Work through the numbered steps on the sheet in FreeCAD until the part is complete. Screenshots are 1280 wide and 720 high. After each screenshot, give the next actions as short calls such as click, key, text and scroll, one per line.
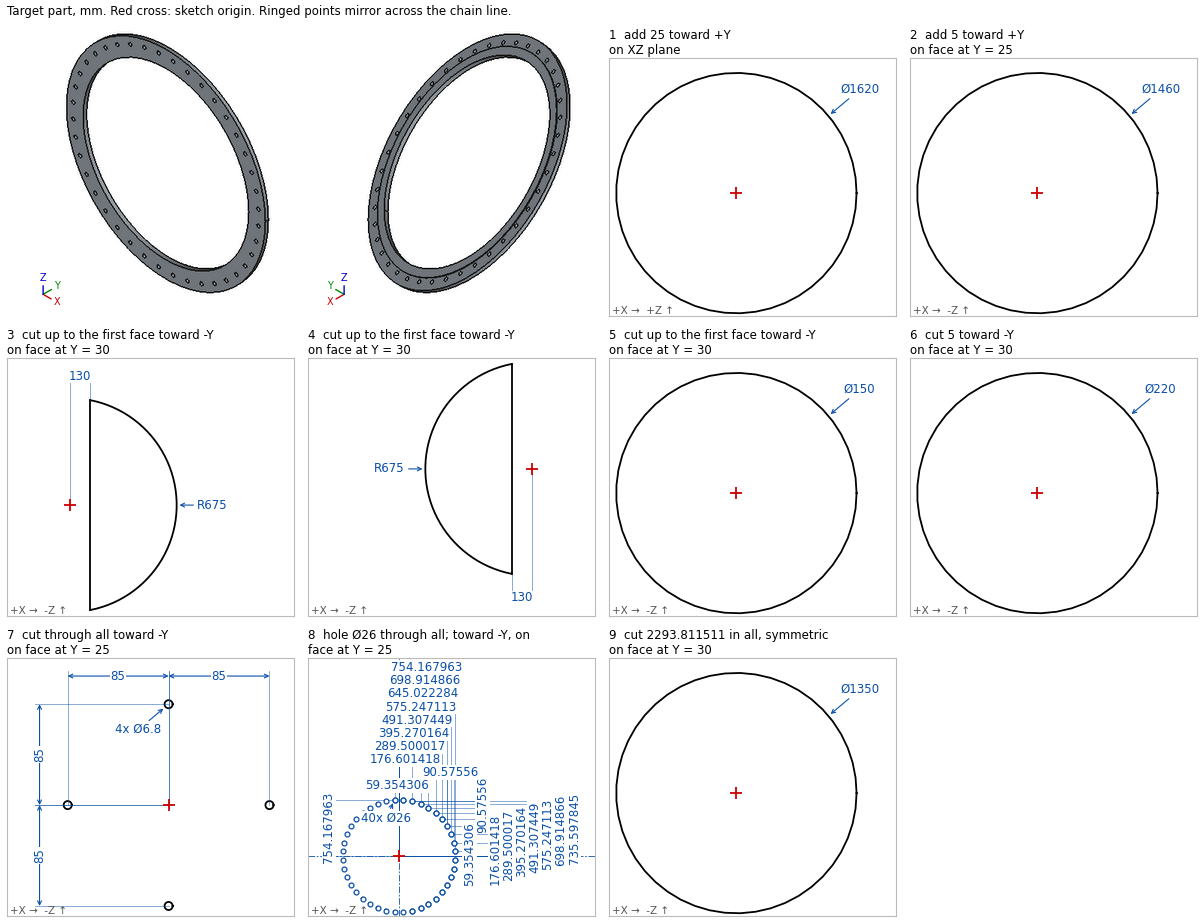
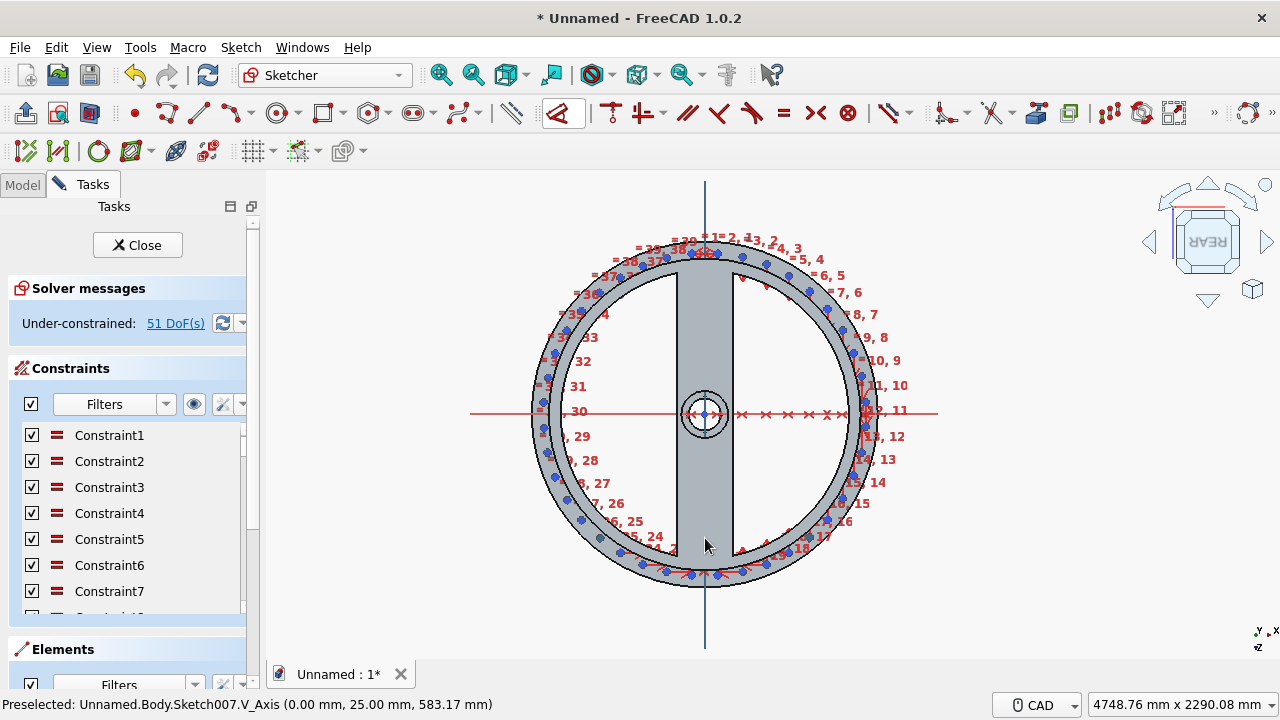
click(816, 114)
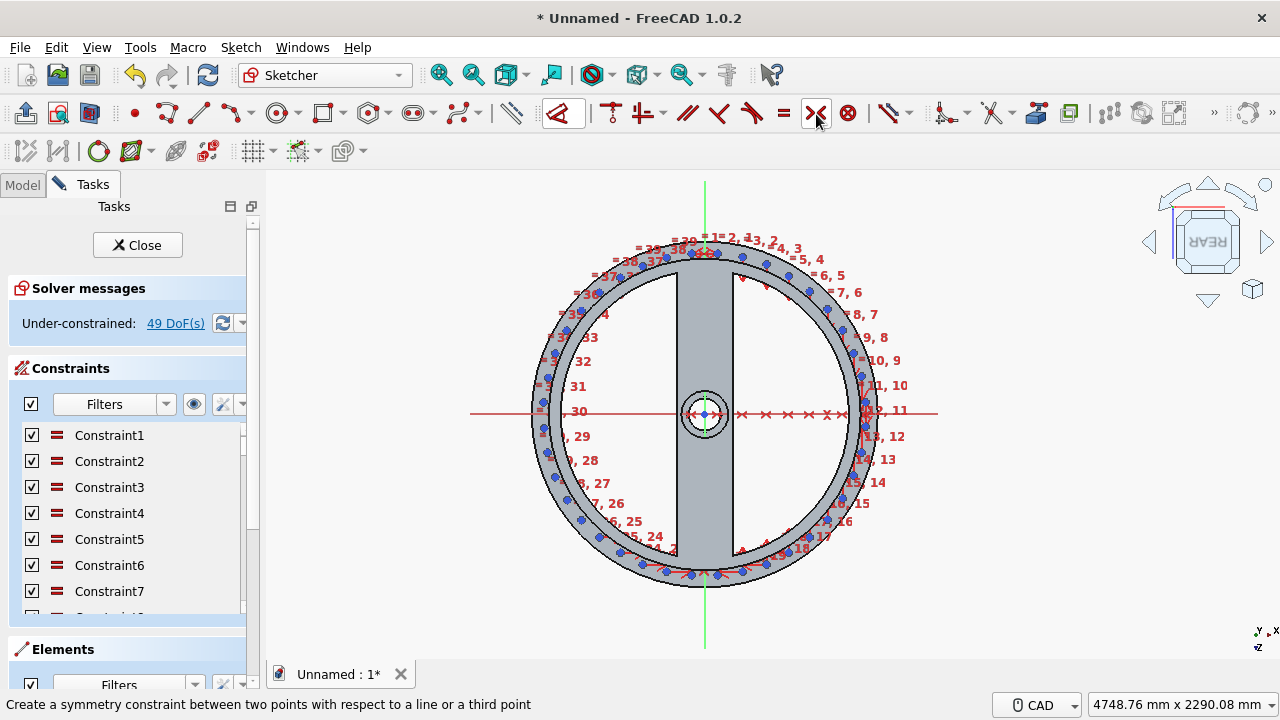
click(828, 520)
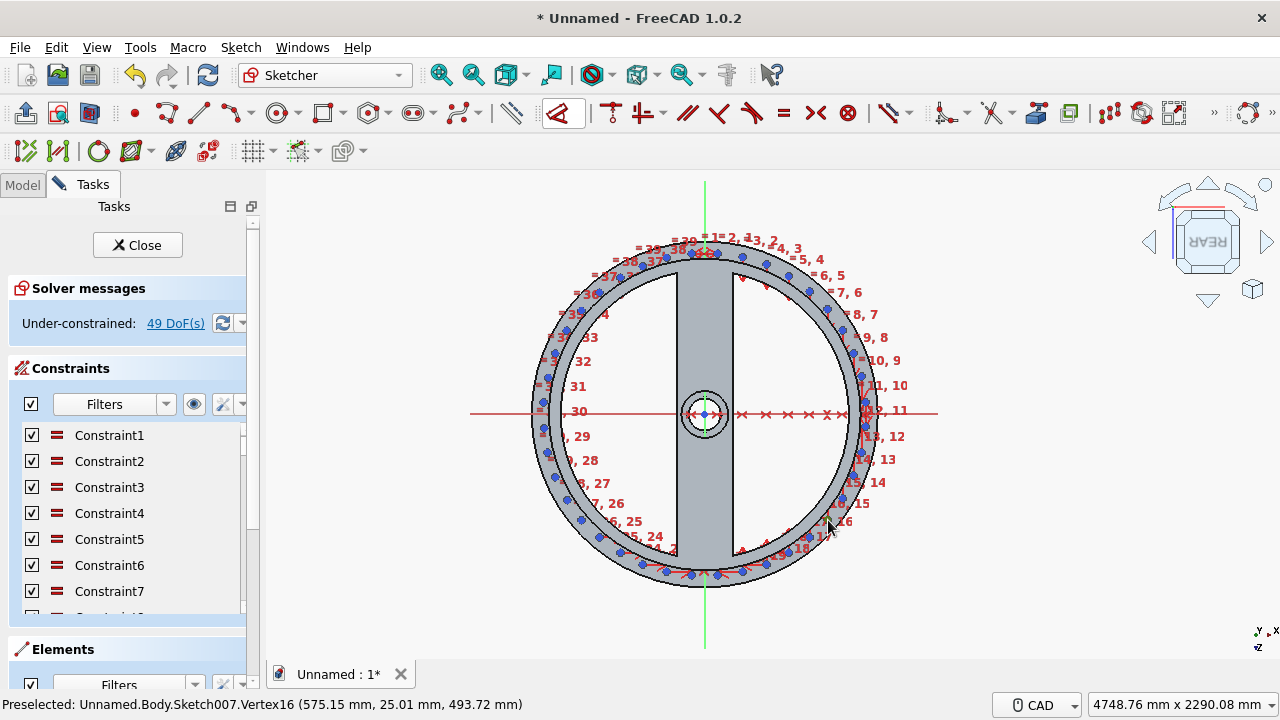
click(582, 520)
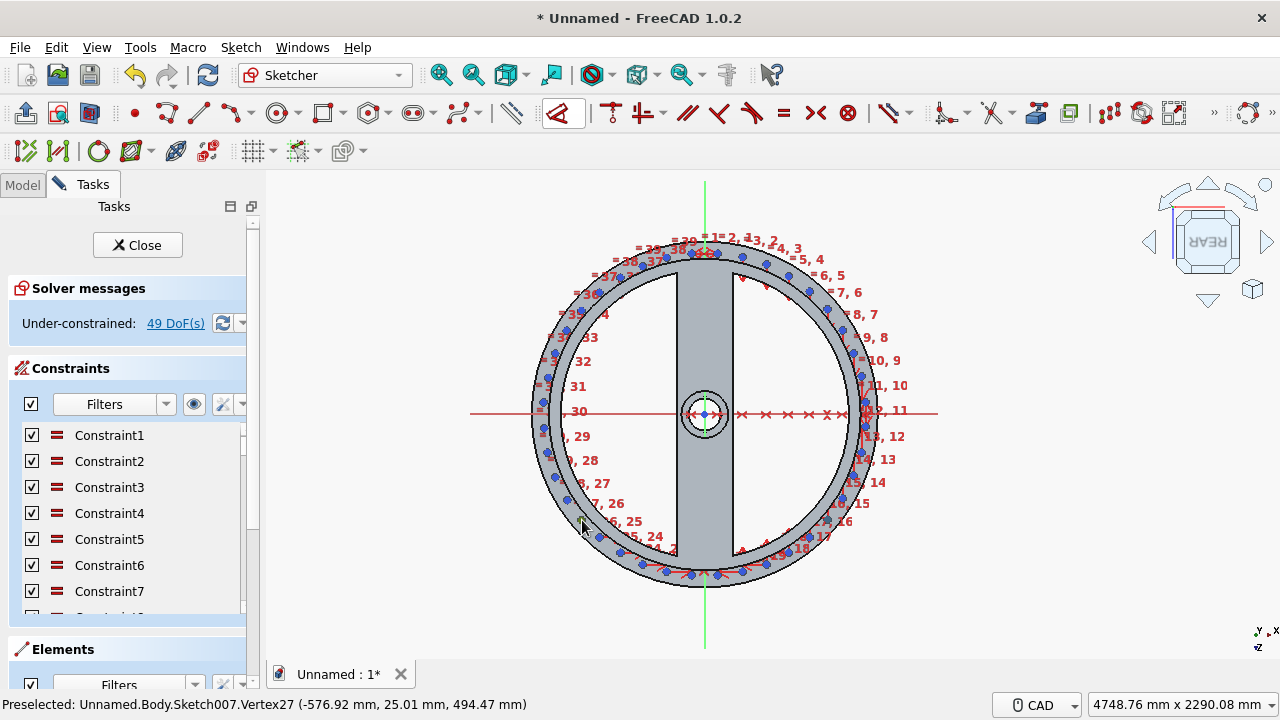
click(705, 507)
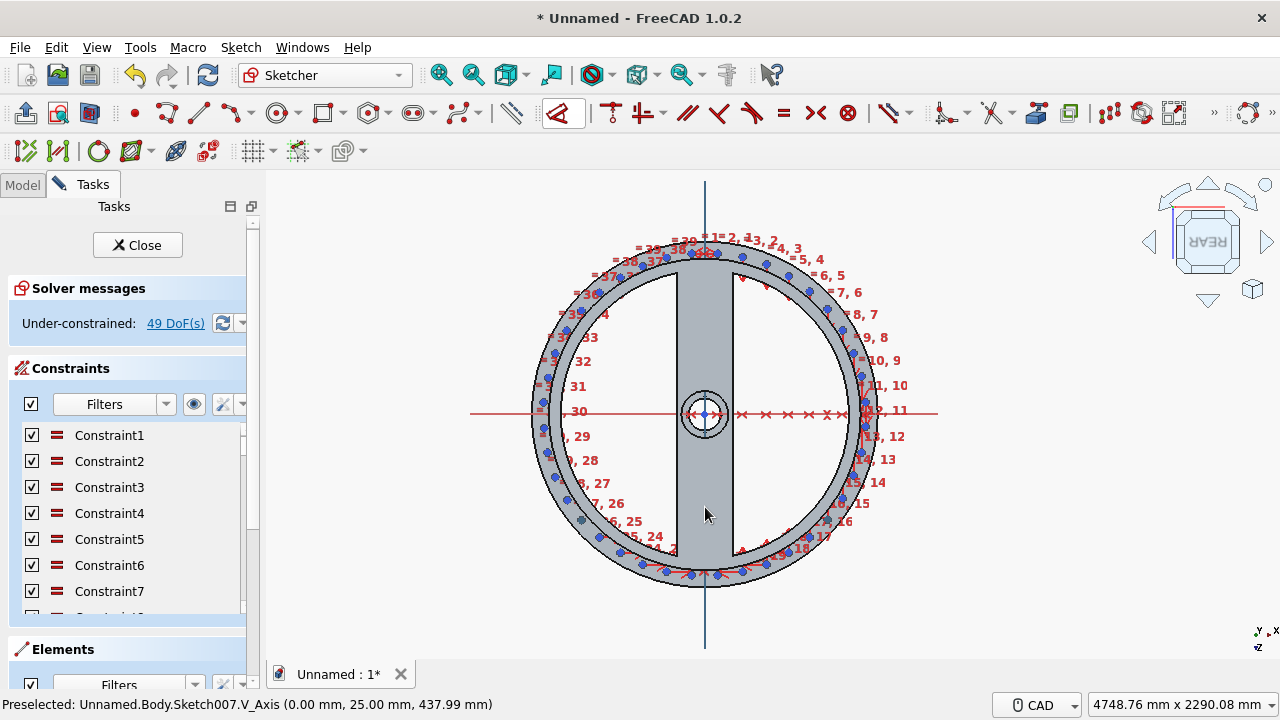
click(816, 114)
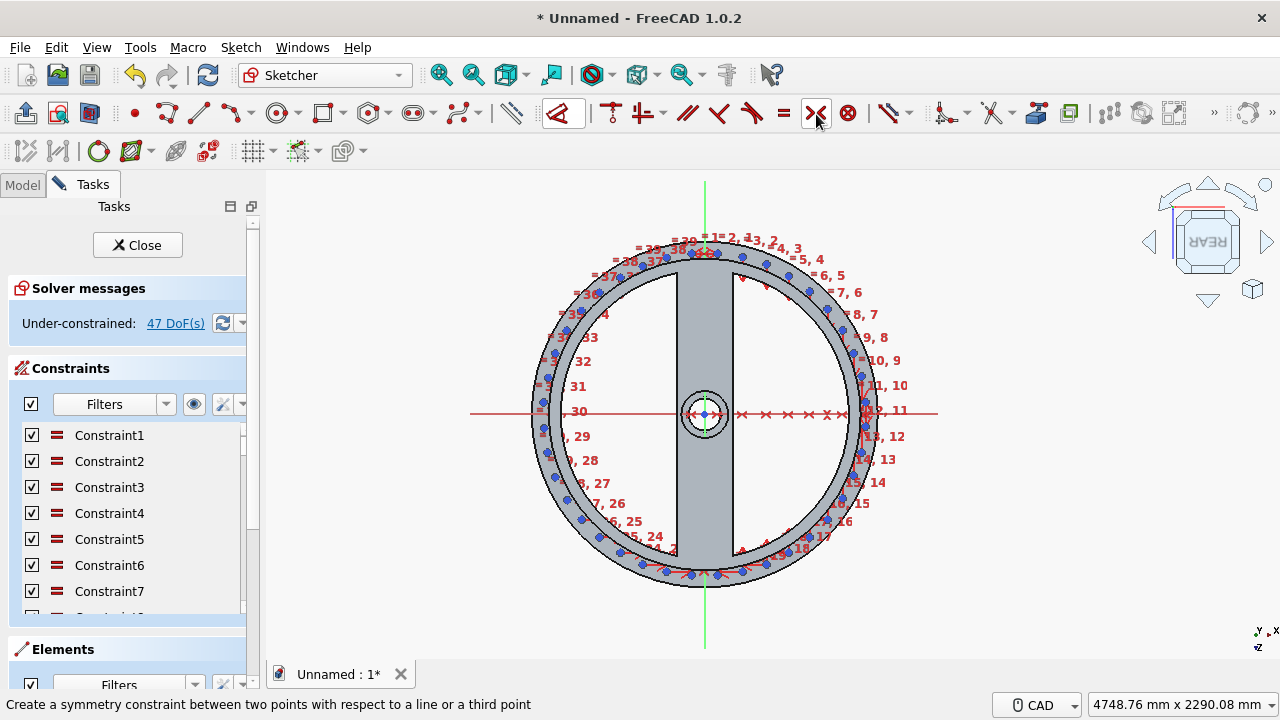
click(843, 499)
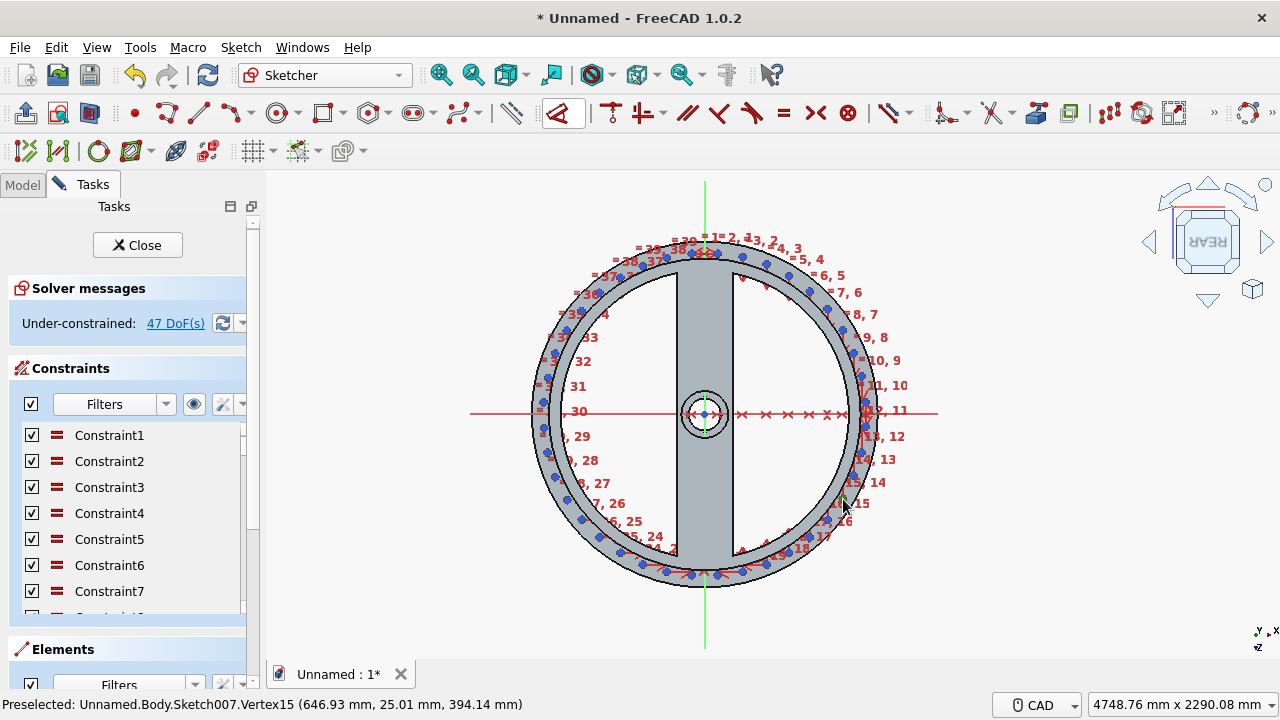
click(567, 500)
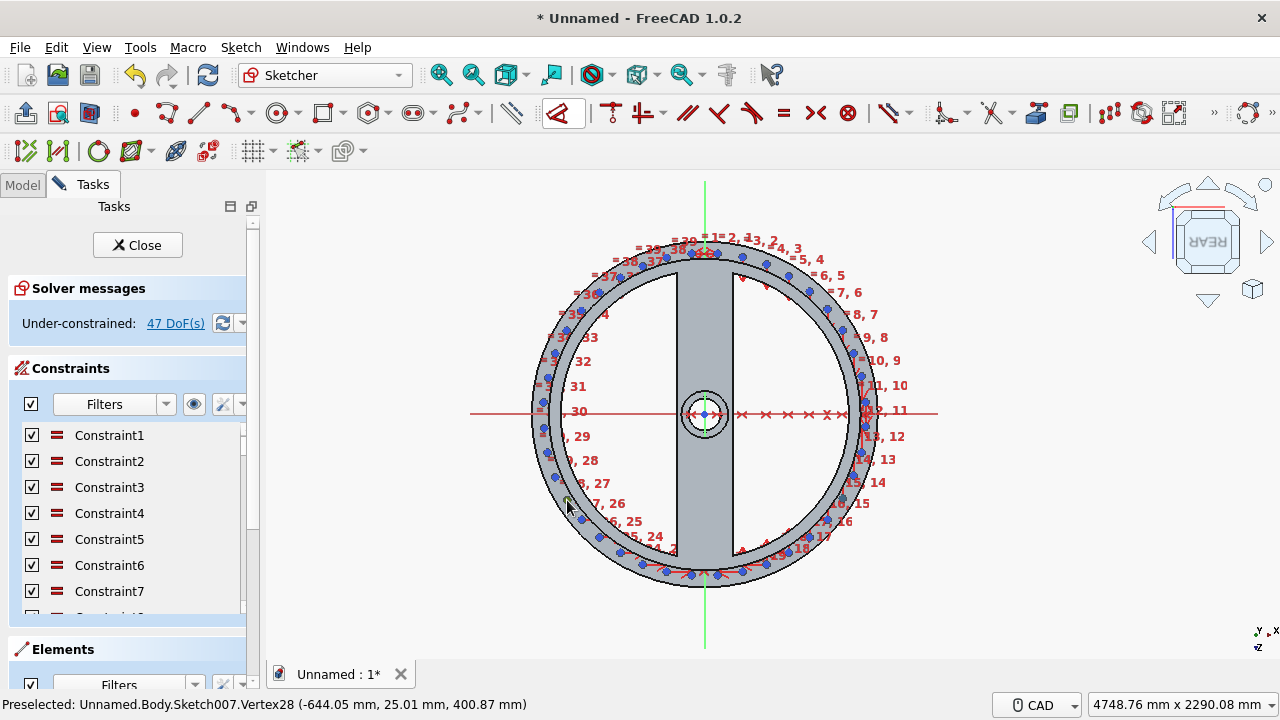
click(705, 507)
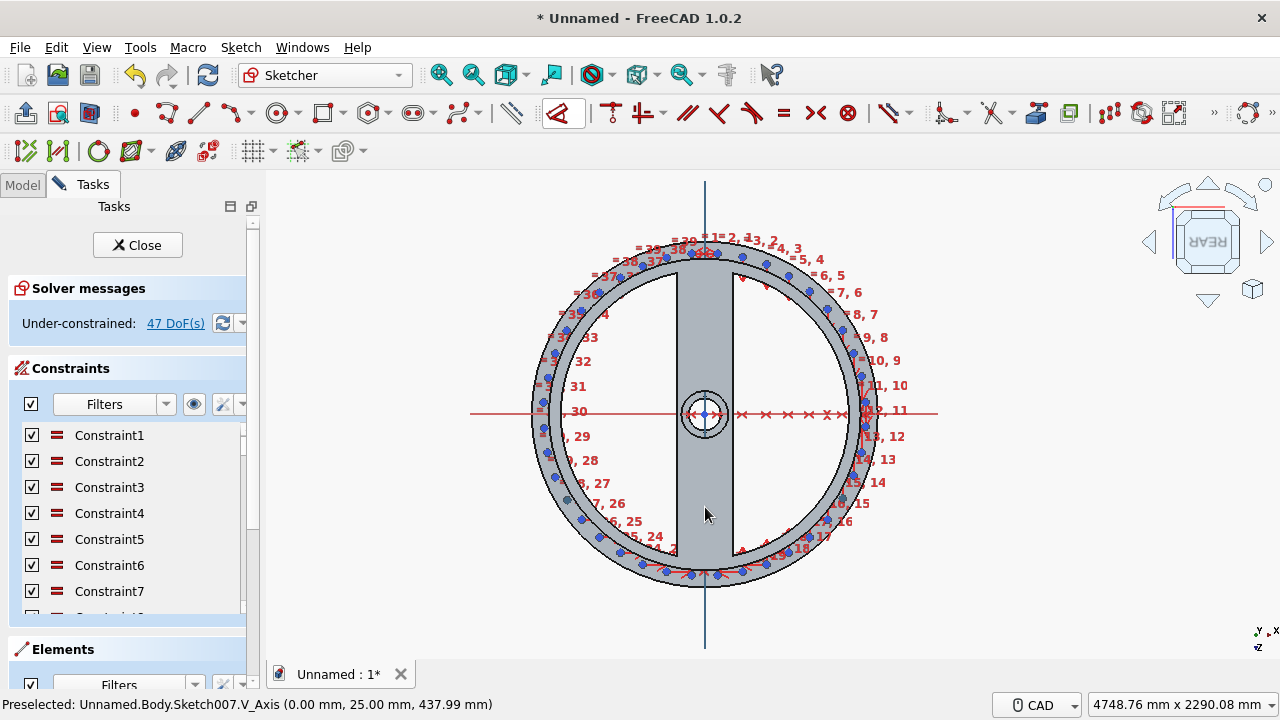
click(816, 114)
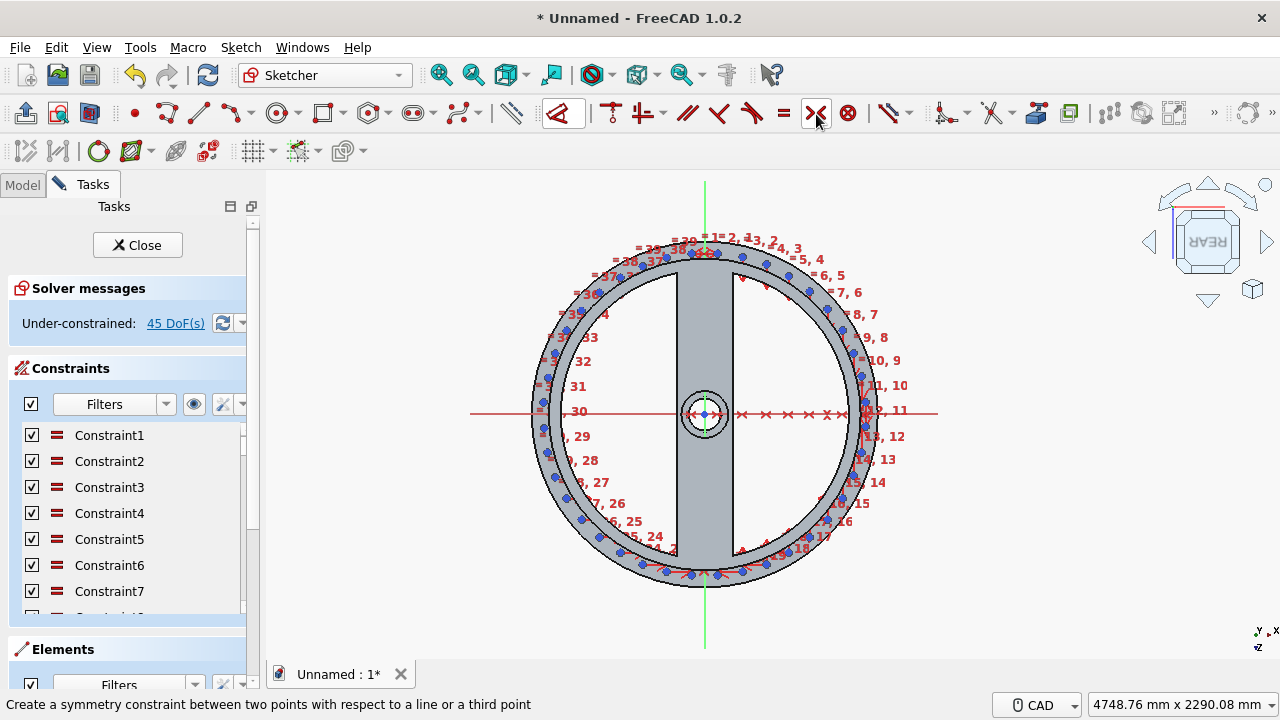
click(854, 476)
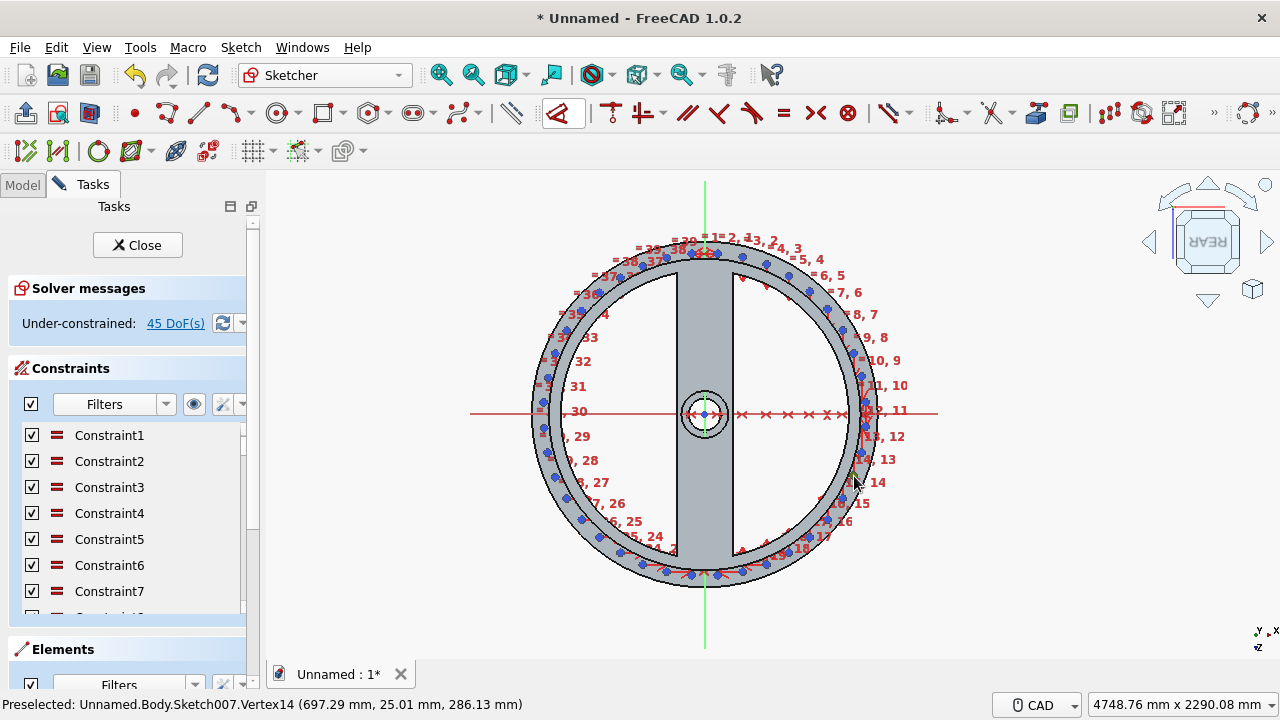
click(555, 477)